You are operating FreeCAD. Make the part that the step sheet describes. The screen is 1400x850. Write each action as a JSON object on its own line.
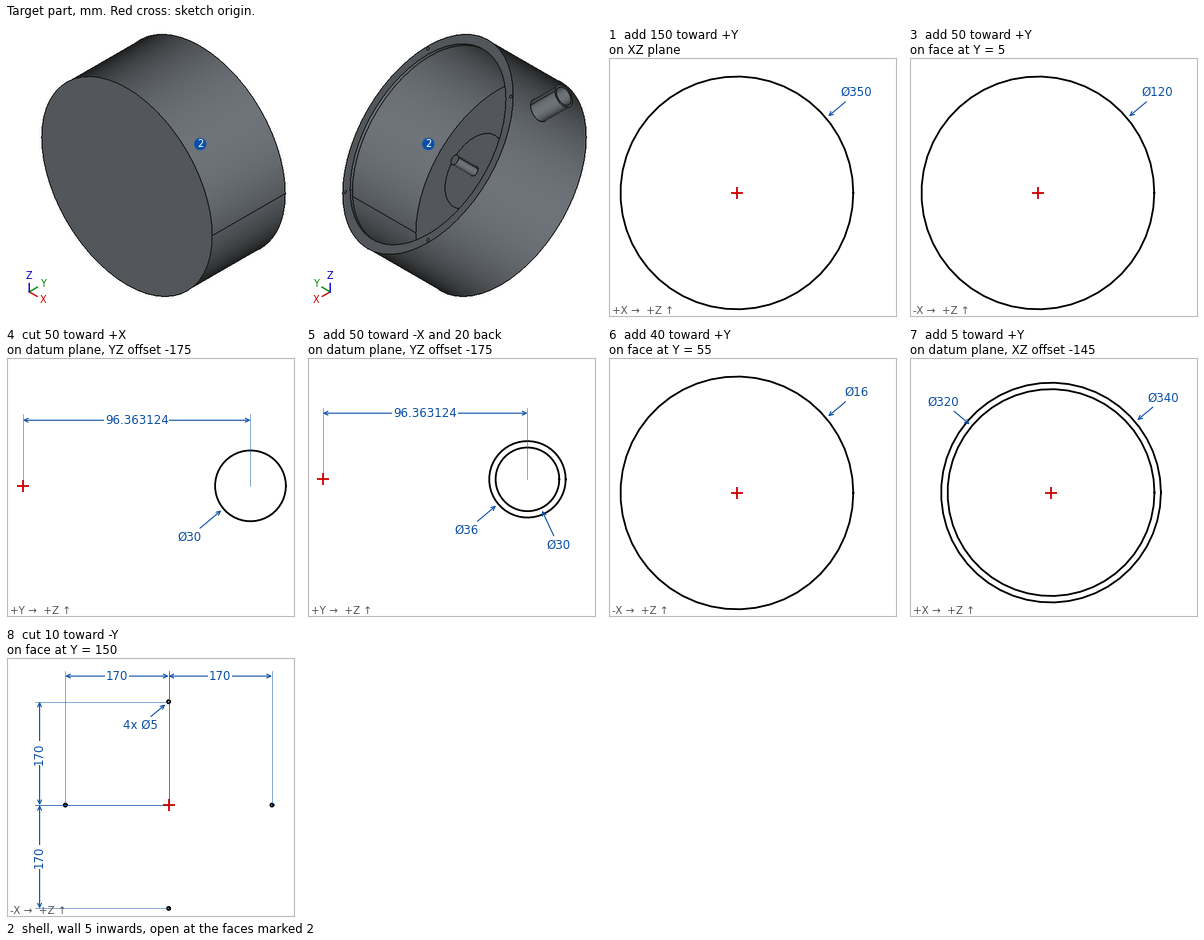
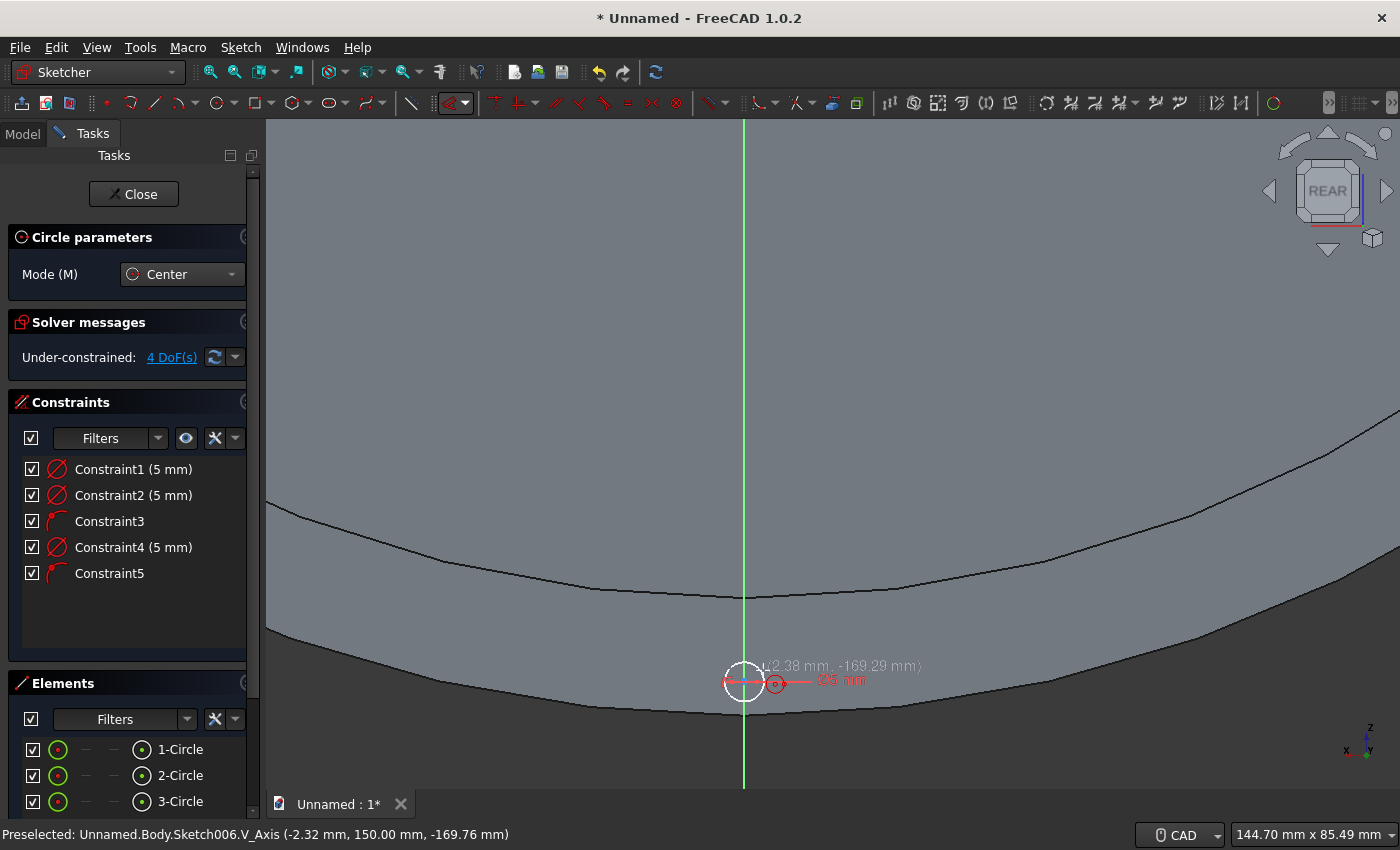
{"action": "scroll", "coordinate": [768, 674], "scroll_direction": "down", "scroll_amount": 9}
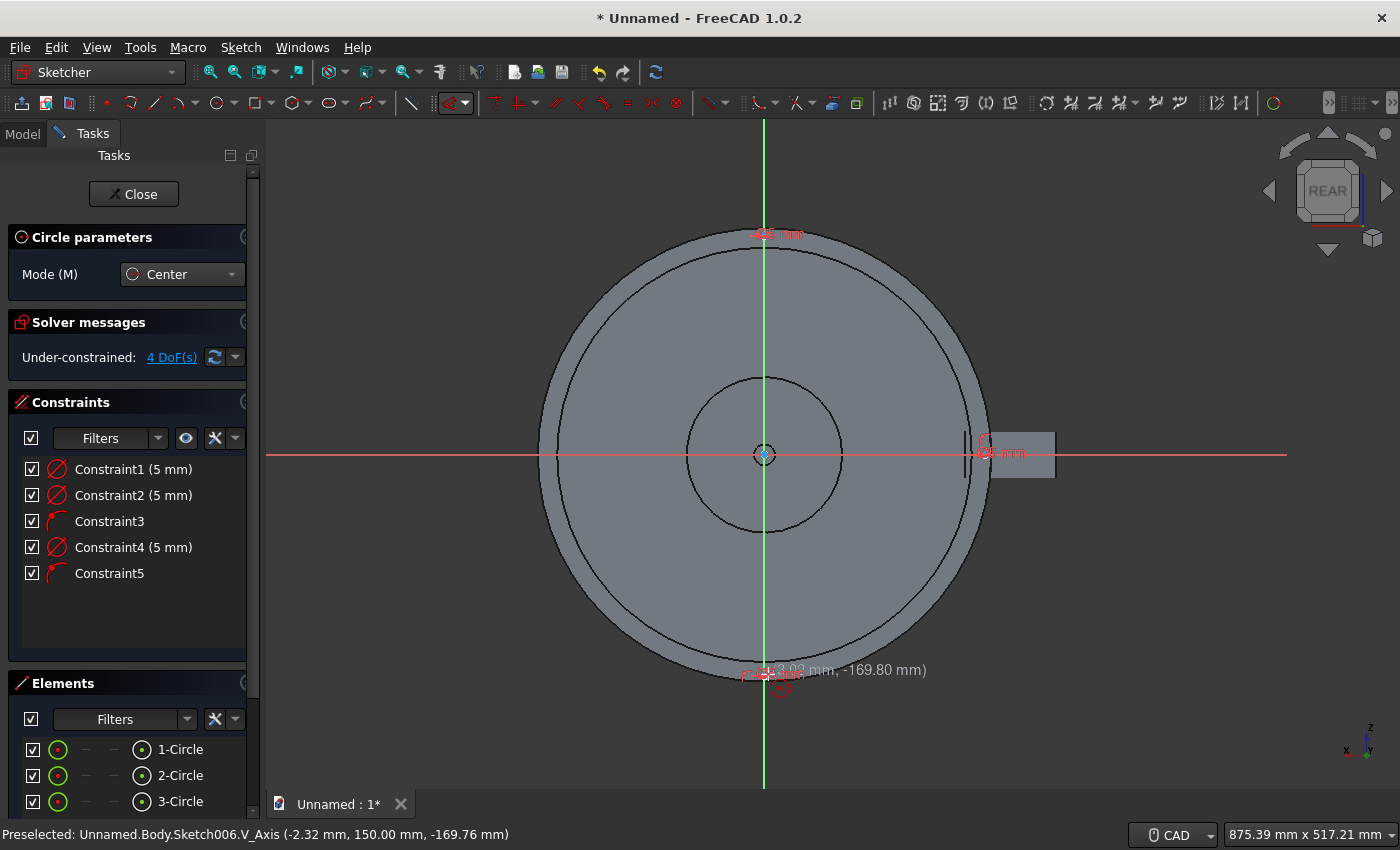
{"action": "scroll", "coordinate": [544, 455], "scroll_direction": "up", "scroll_amount": 10}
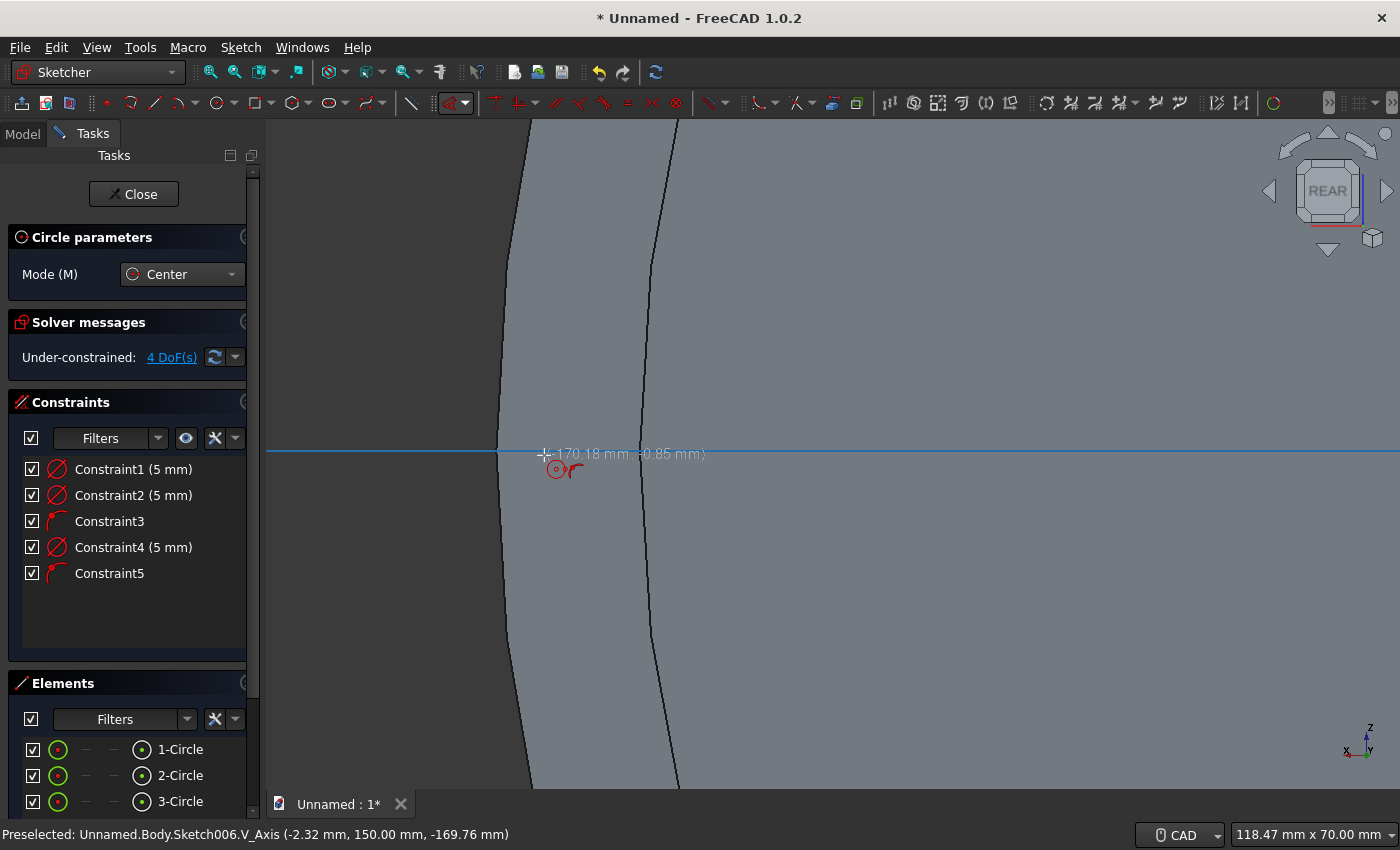
{"action": "scroll", "coordinate": [544, 454], "scroll_direction": "down", "scroll_amount": 10}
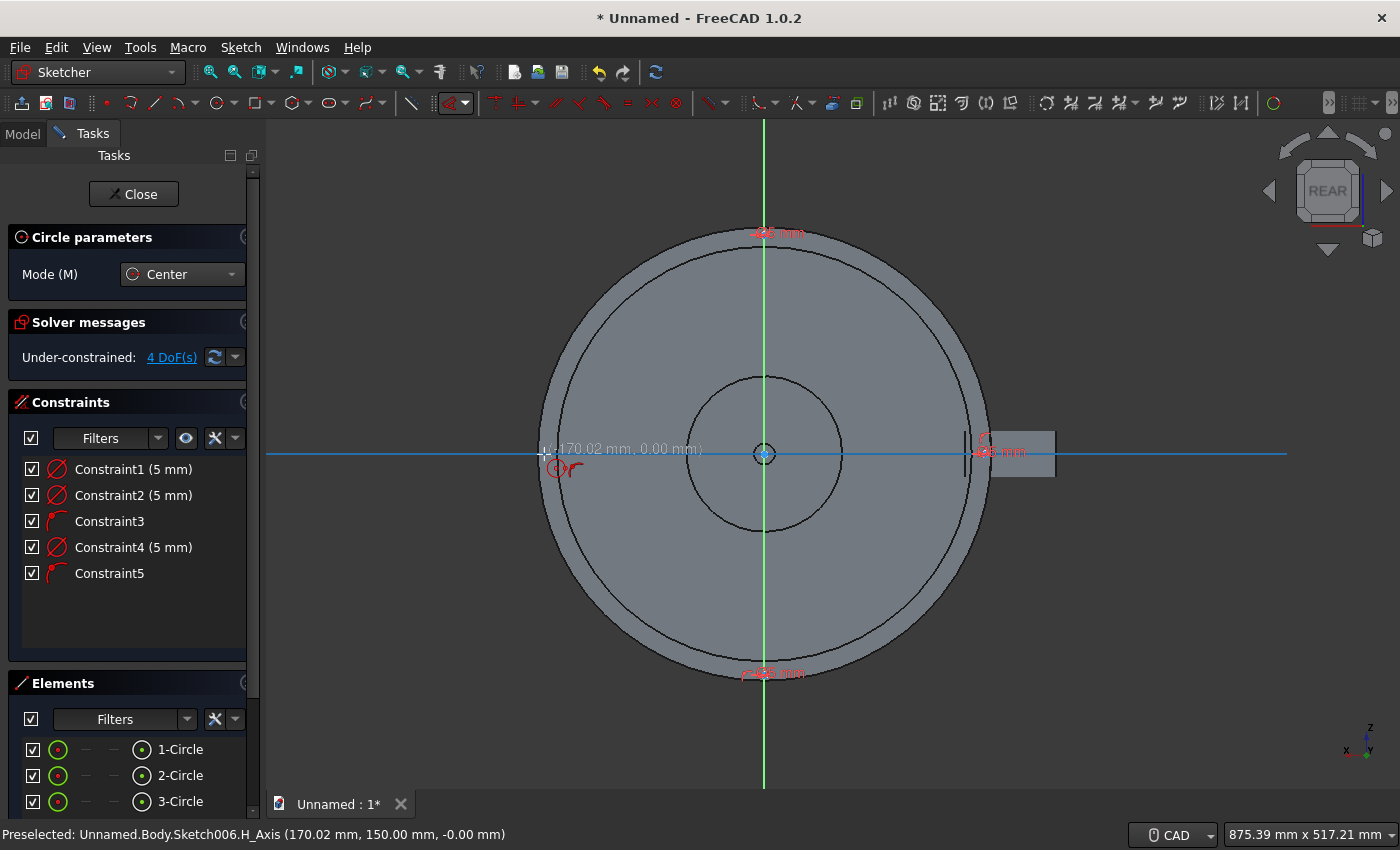
{"action": "left_click", "coordinate": [544, 454]}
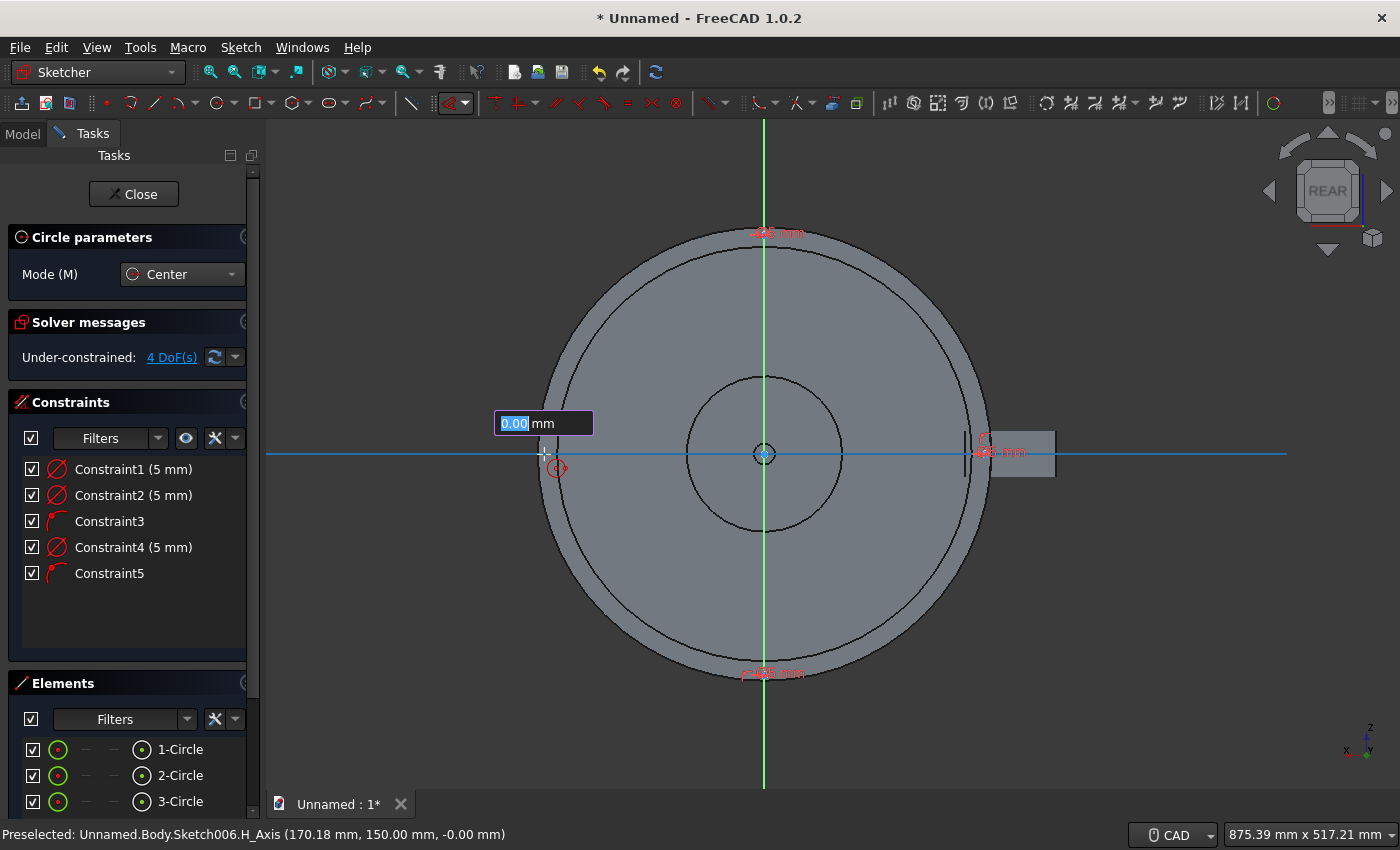
{"action": "scroll", "coordinate": [543, 457], "scroll_direction": "up", "scroll_amount": 9}
{"action": "mouse_move", "coordinate": [543, 455]}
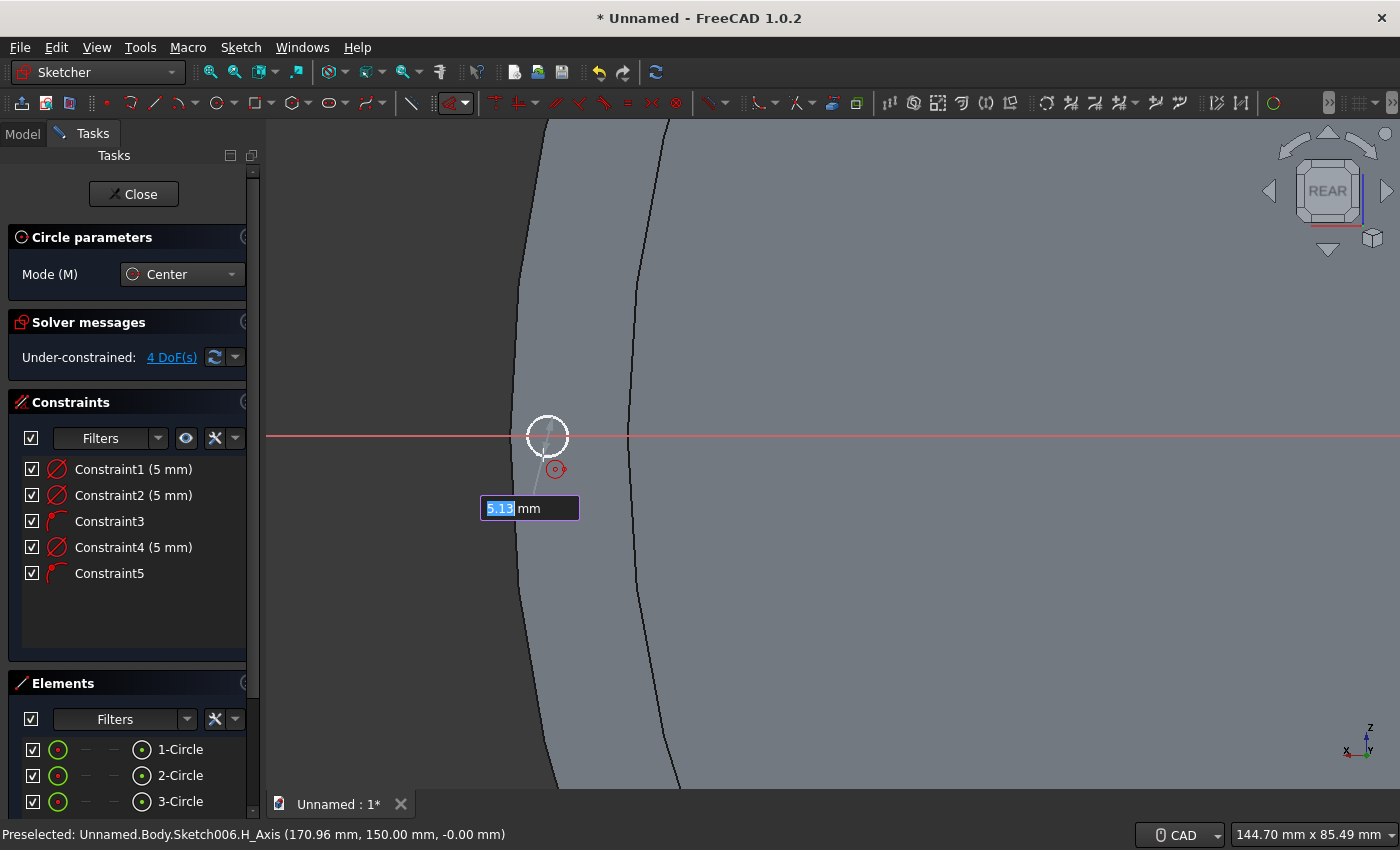
{"action": "type", "text": "5"}
{"action": "key", "text": "Return"}
{"action": "key", "text": "Escape"}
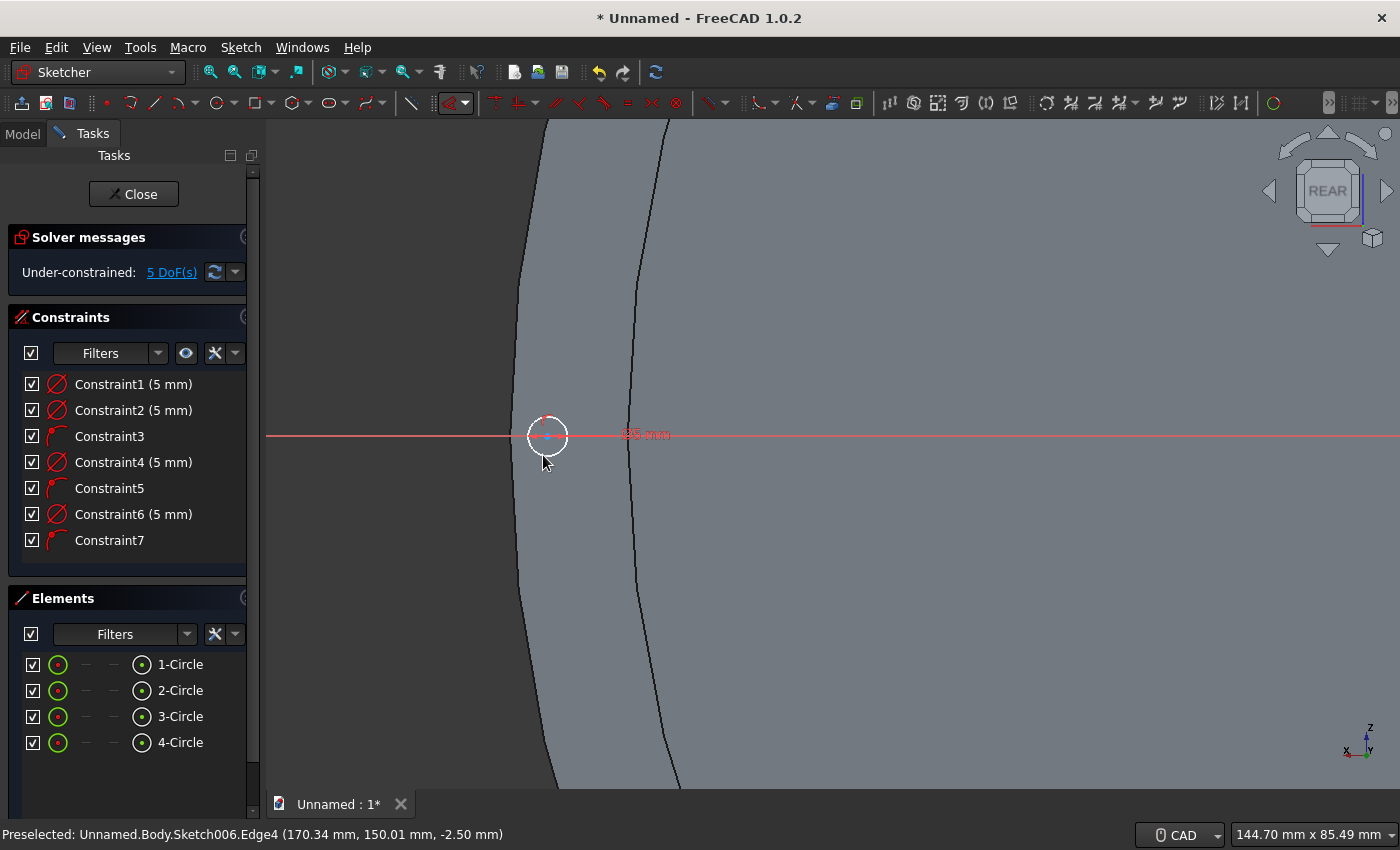
{"action": "scroll", "coordinate": [543, 457], "scroll_direction": "down", "scroll_amount": 9}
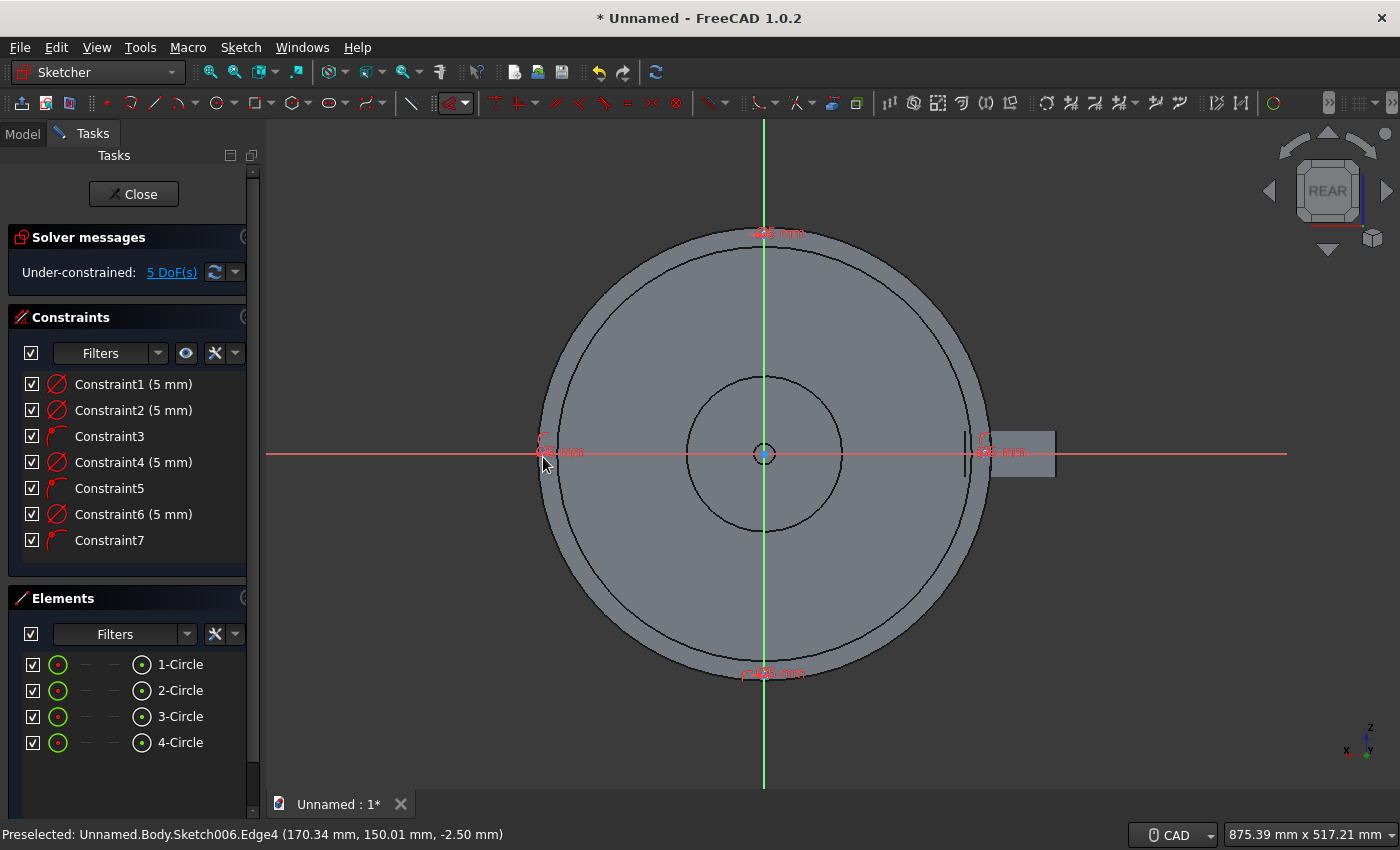
{"action": "left_click", "coordinate": [764, 235]}